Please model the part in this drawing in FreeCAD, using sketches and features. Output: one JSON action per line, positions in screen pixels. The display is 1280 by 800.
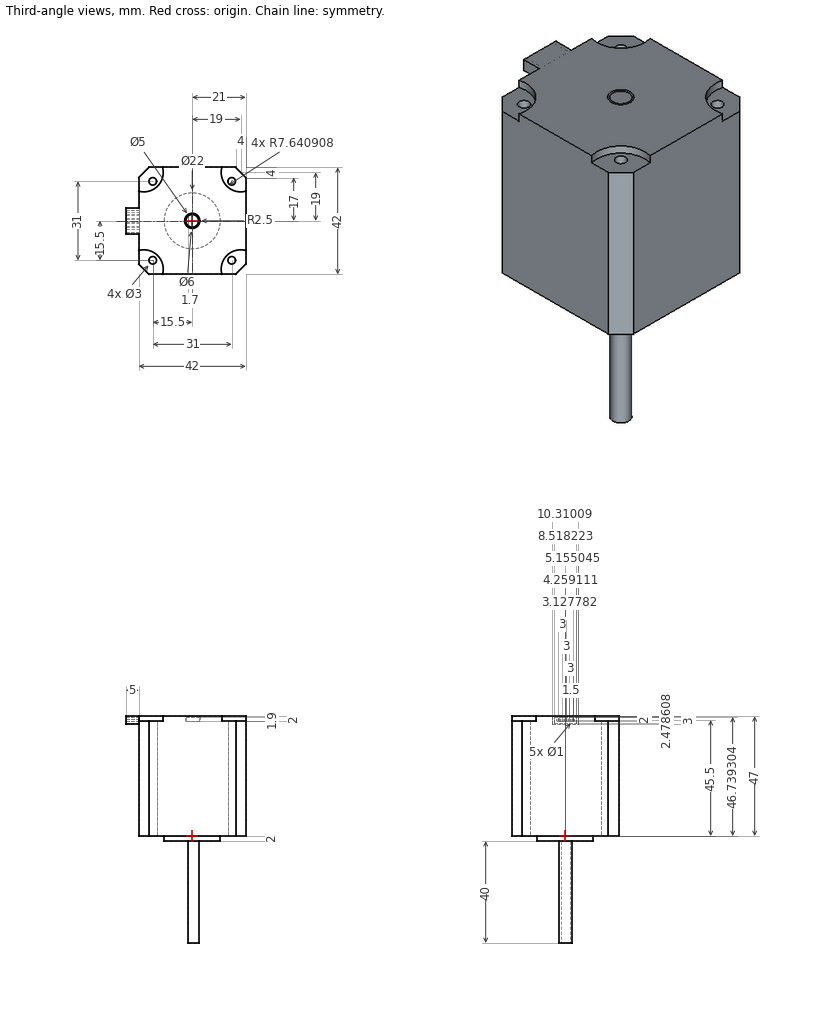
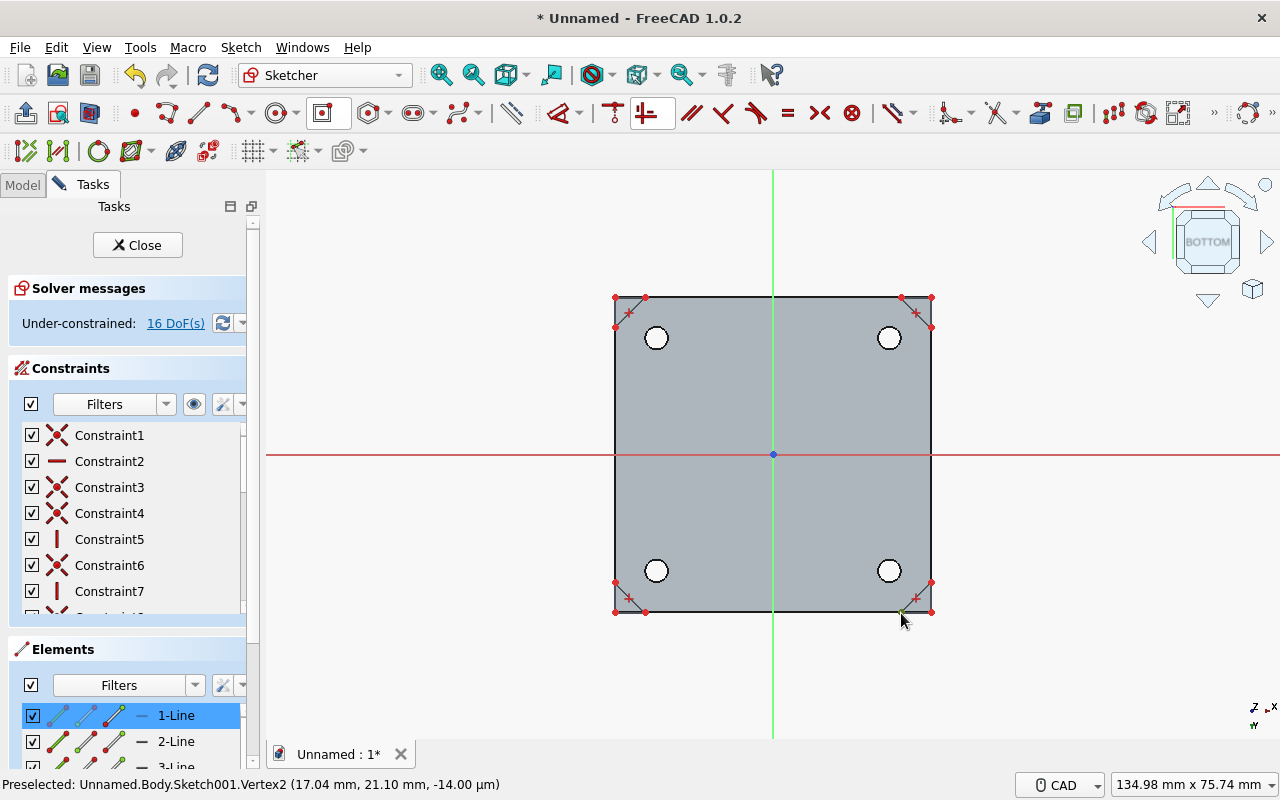
{"action": "left_click", "coordinate": [645, 613]}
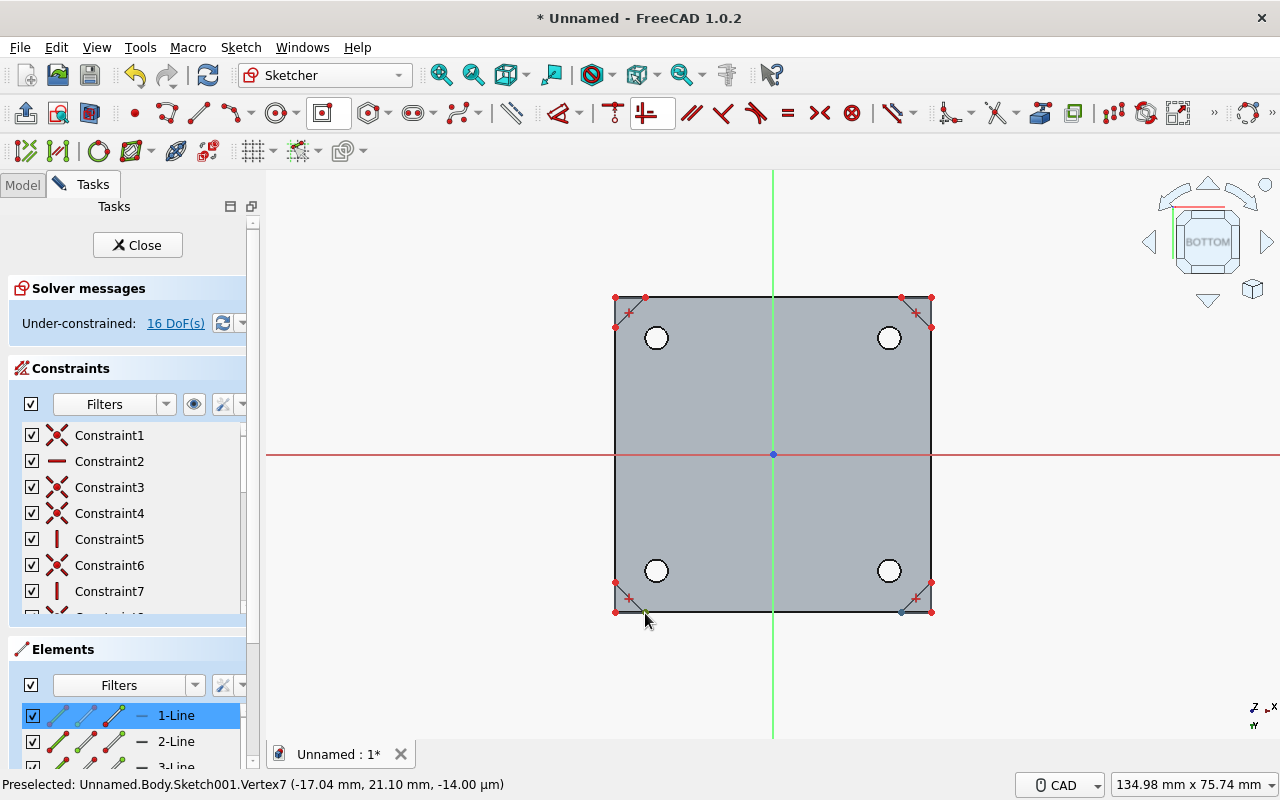
{"action": "left_click", "coordinate": [773, 674]}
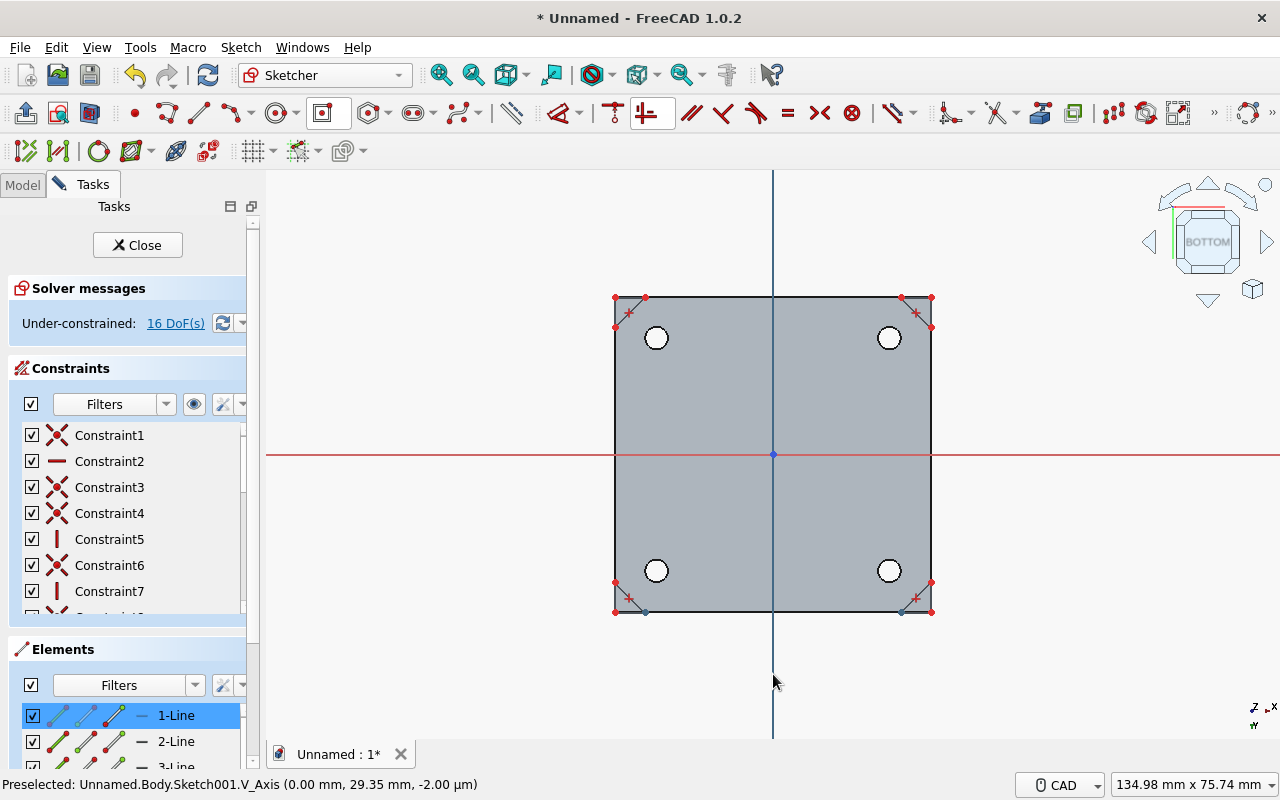
{"action": "left_click", "coordinate": [820, 114]}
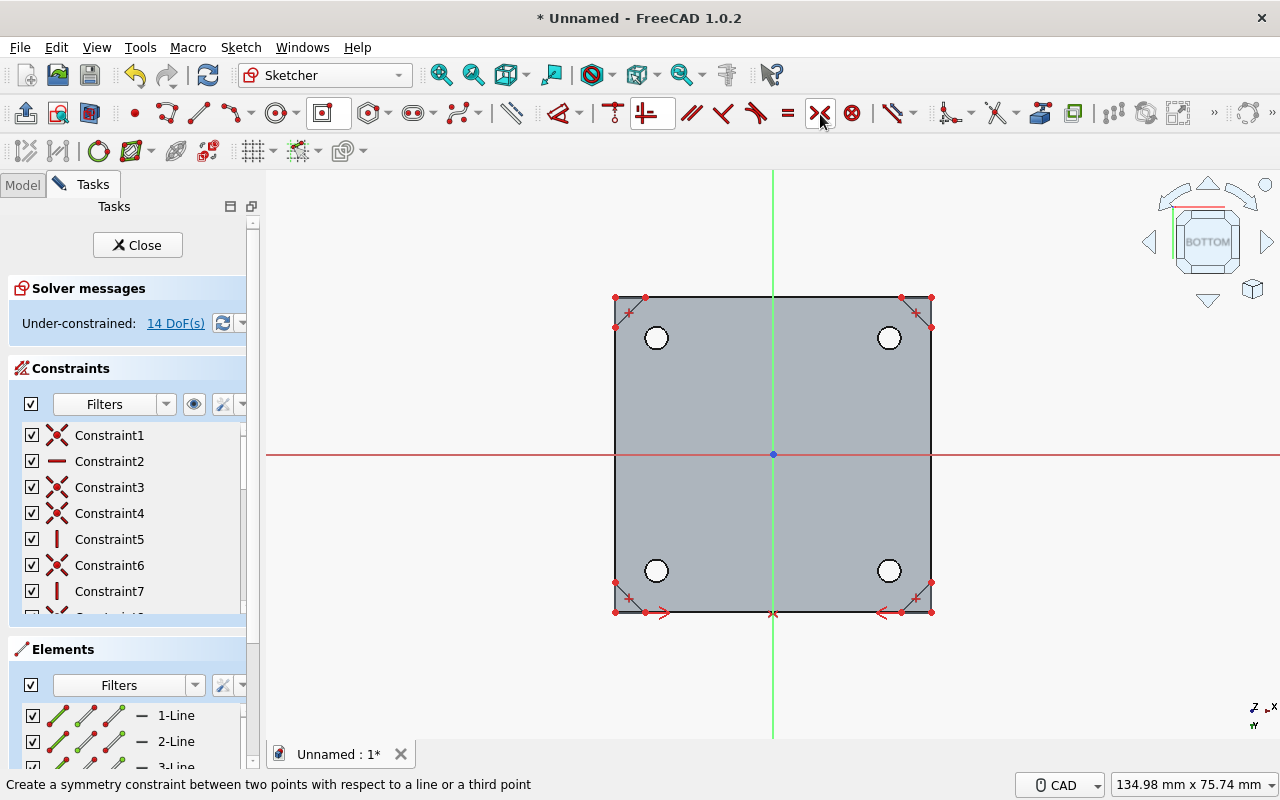
{"action": "left_click", "coordinate": [931, 583]}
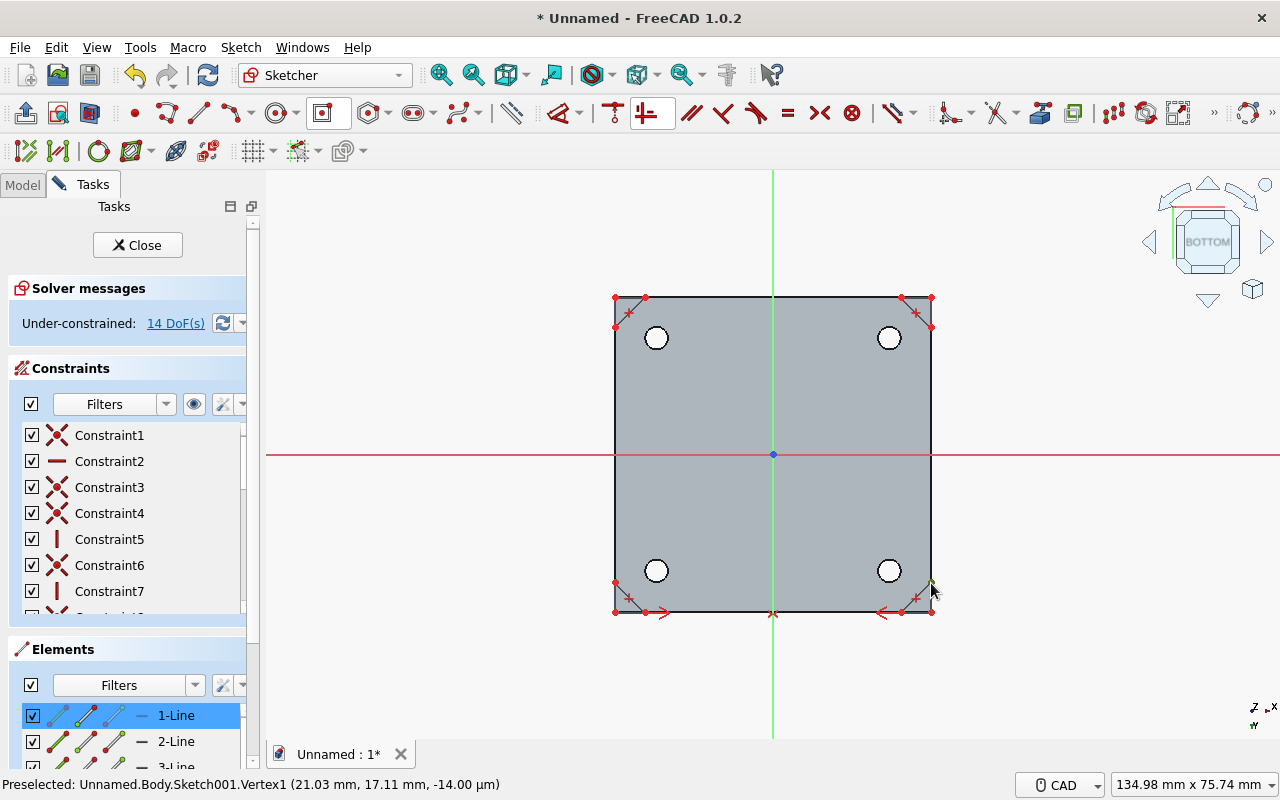
{"action": "left_click", "coordinate": [615, 583]}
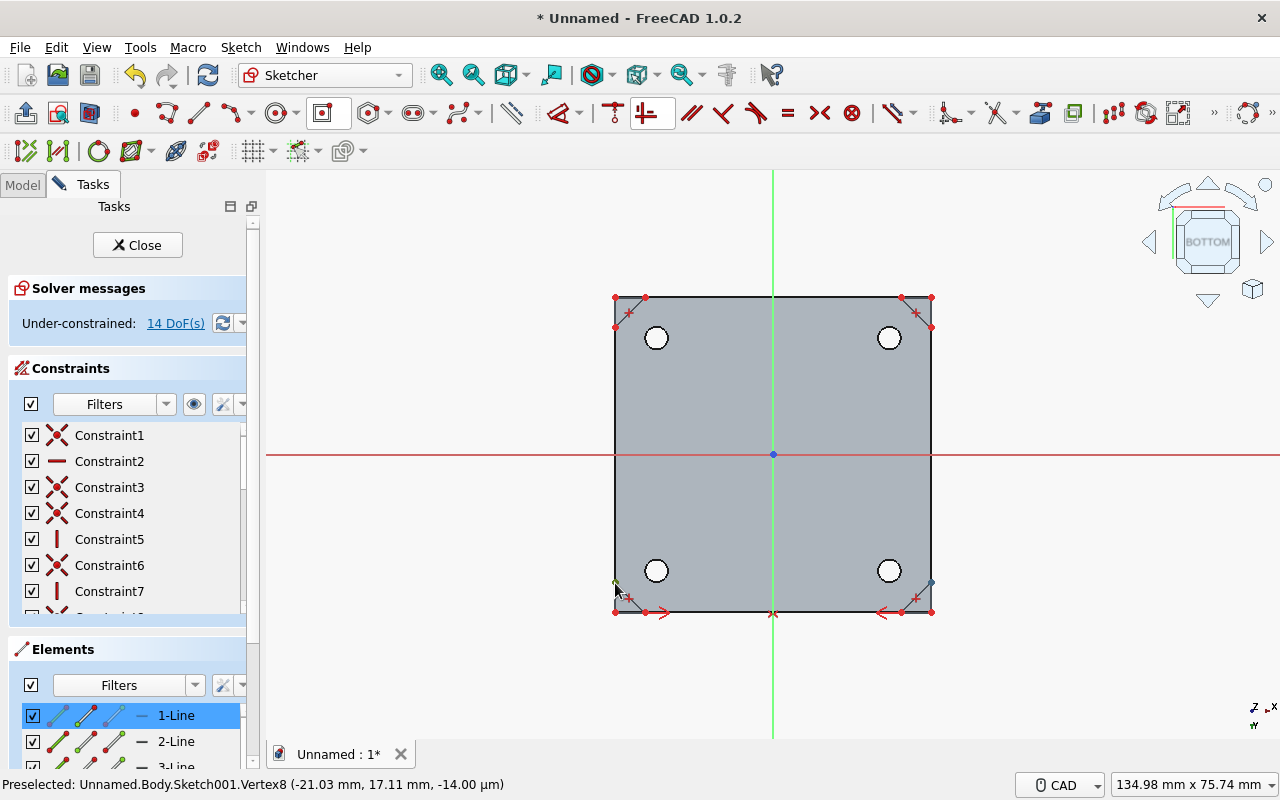
{"action": "left_click", "coordinate": [773, 674]}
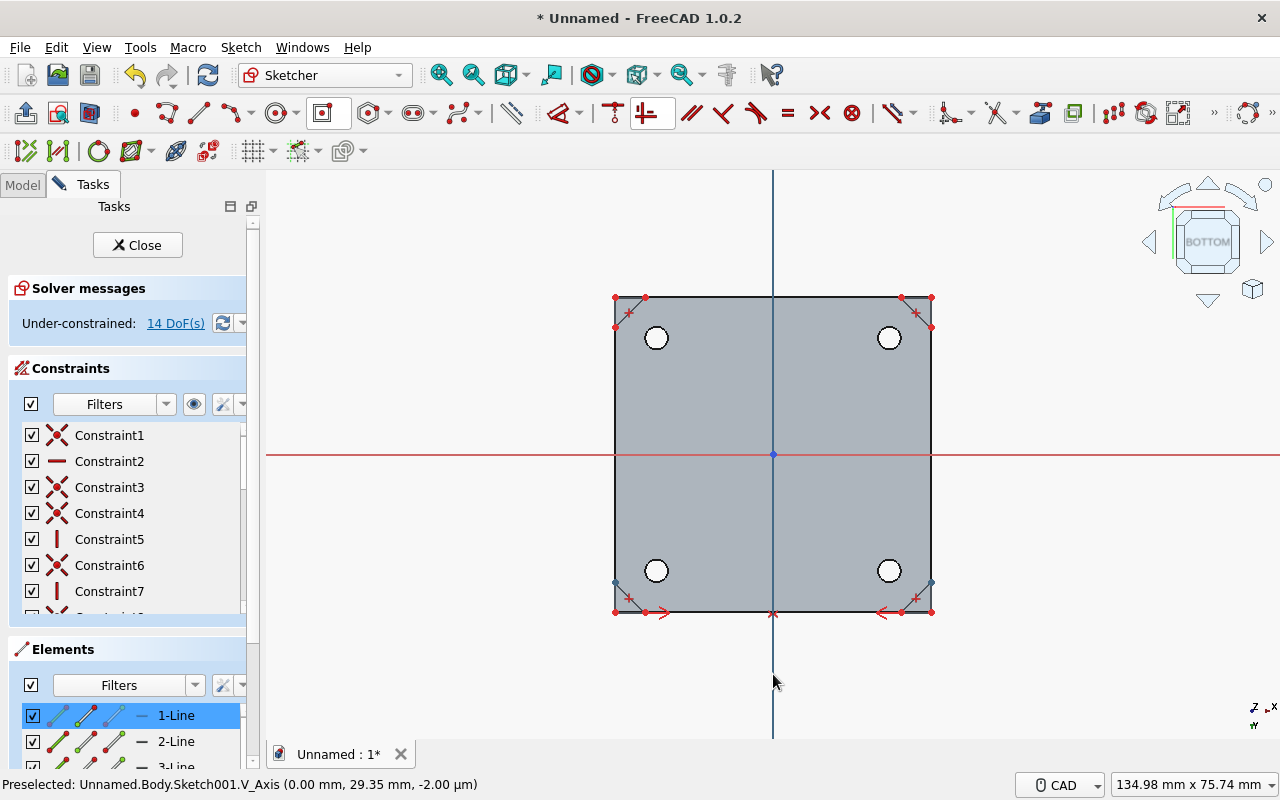
{"action": "left_click", "coordinate": [820, 114]}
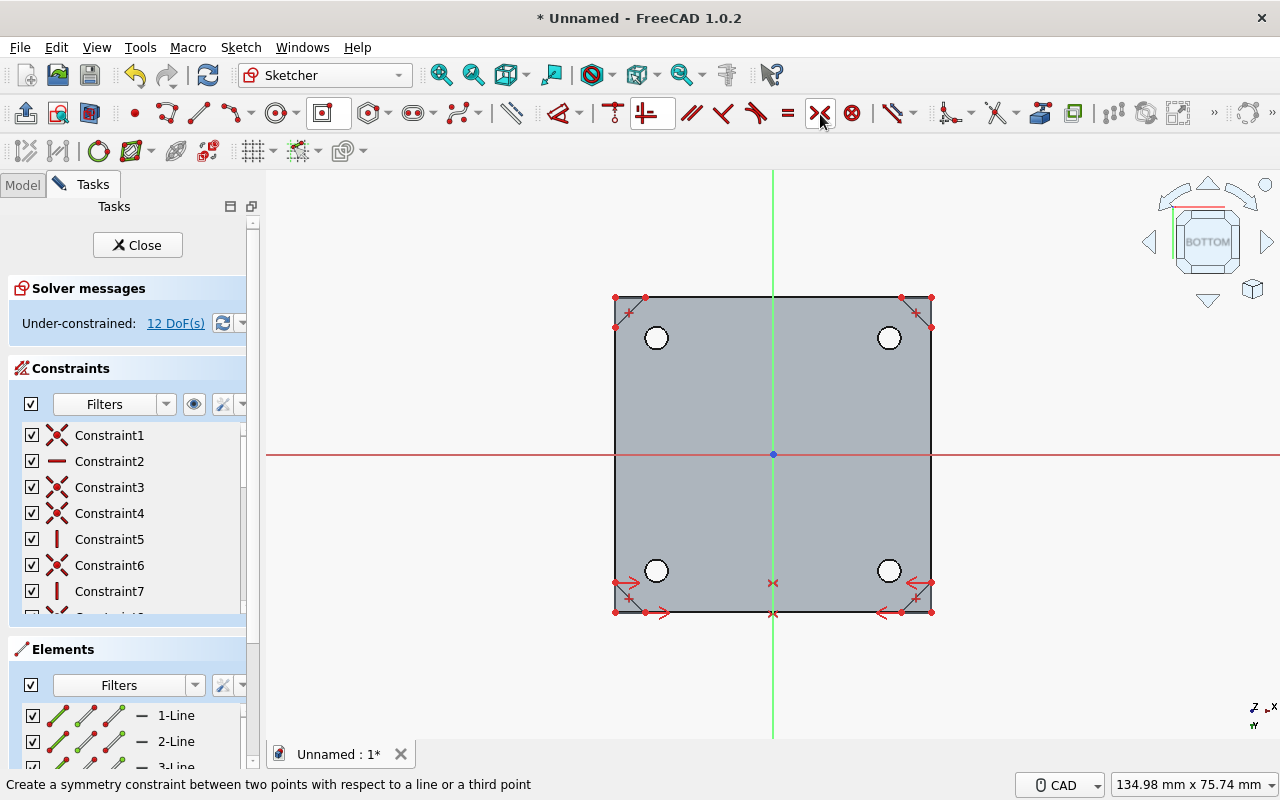
{"action": "left_click", "coordinate": [615, 583]}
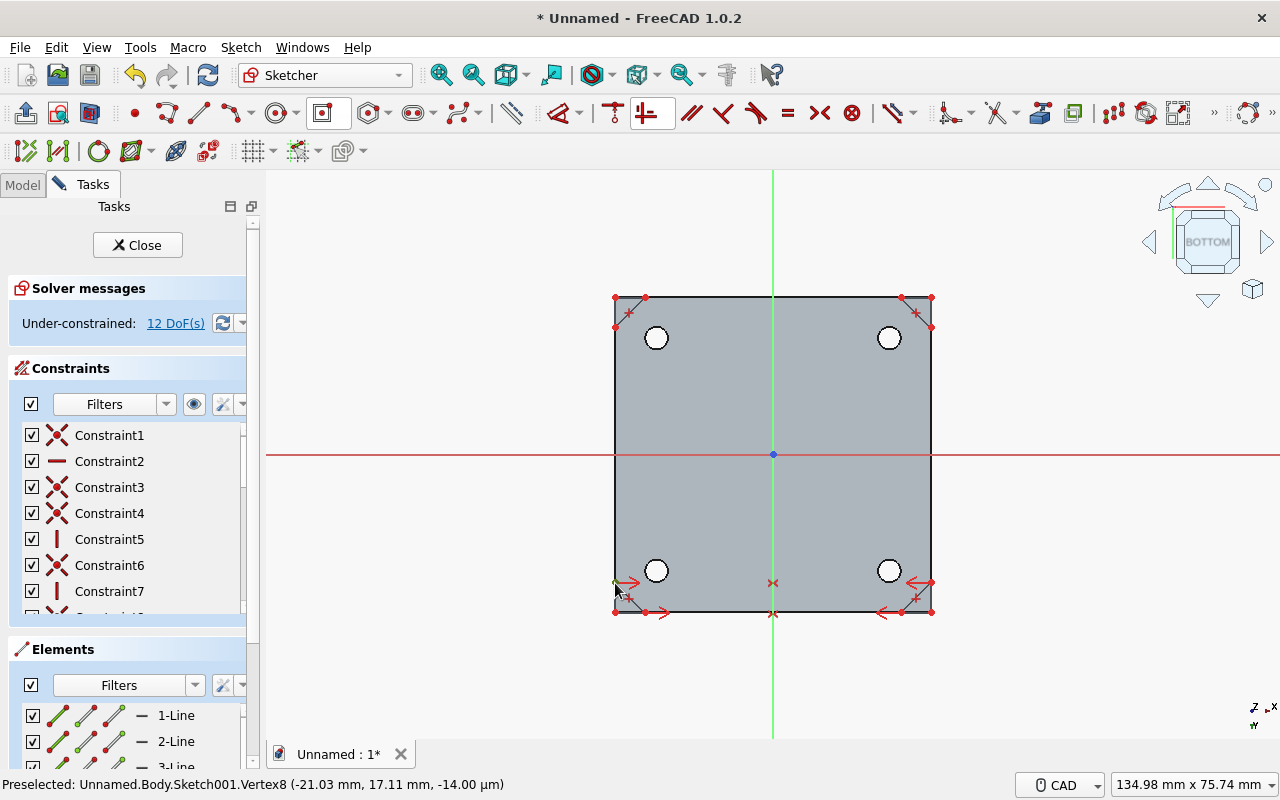
{"action": "left_click", "coordinate": [615, 328]}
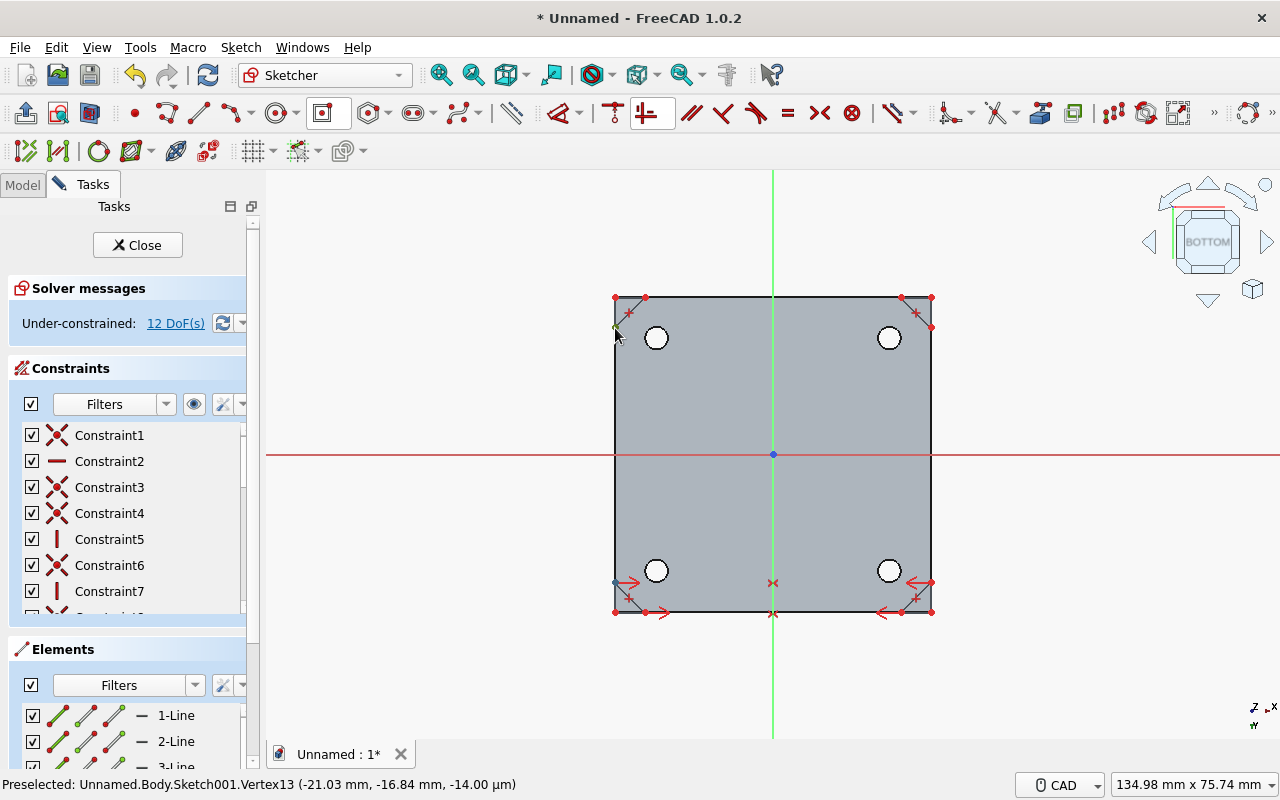
{"action": "left_click", "coordinate": [353, 454]}